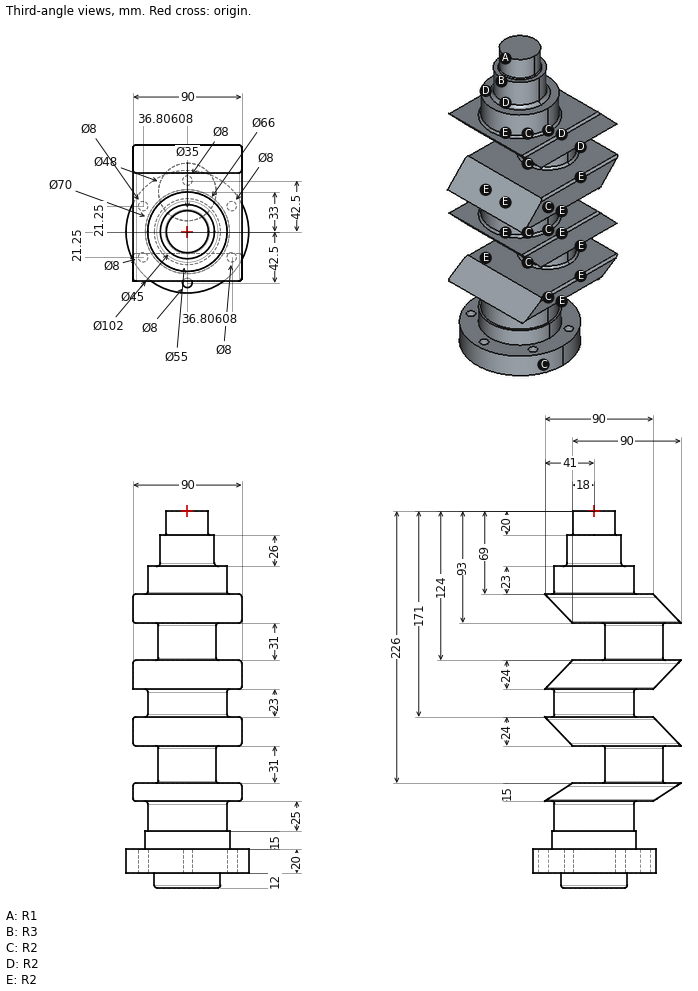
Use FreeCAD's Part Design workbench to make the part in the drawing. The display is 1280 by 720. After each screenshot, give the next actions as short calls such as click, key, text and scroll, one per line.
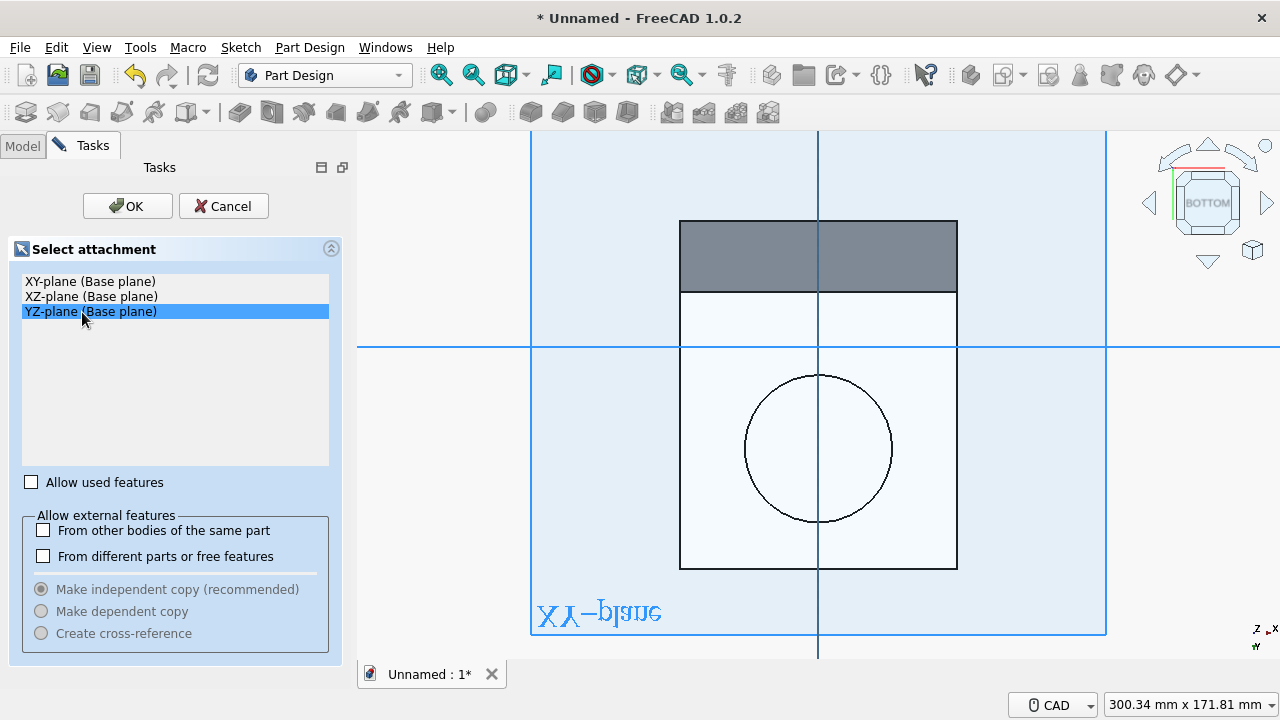
click(128, 206)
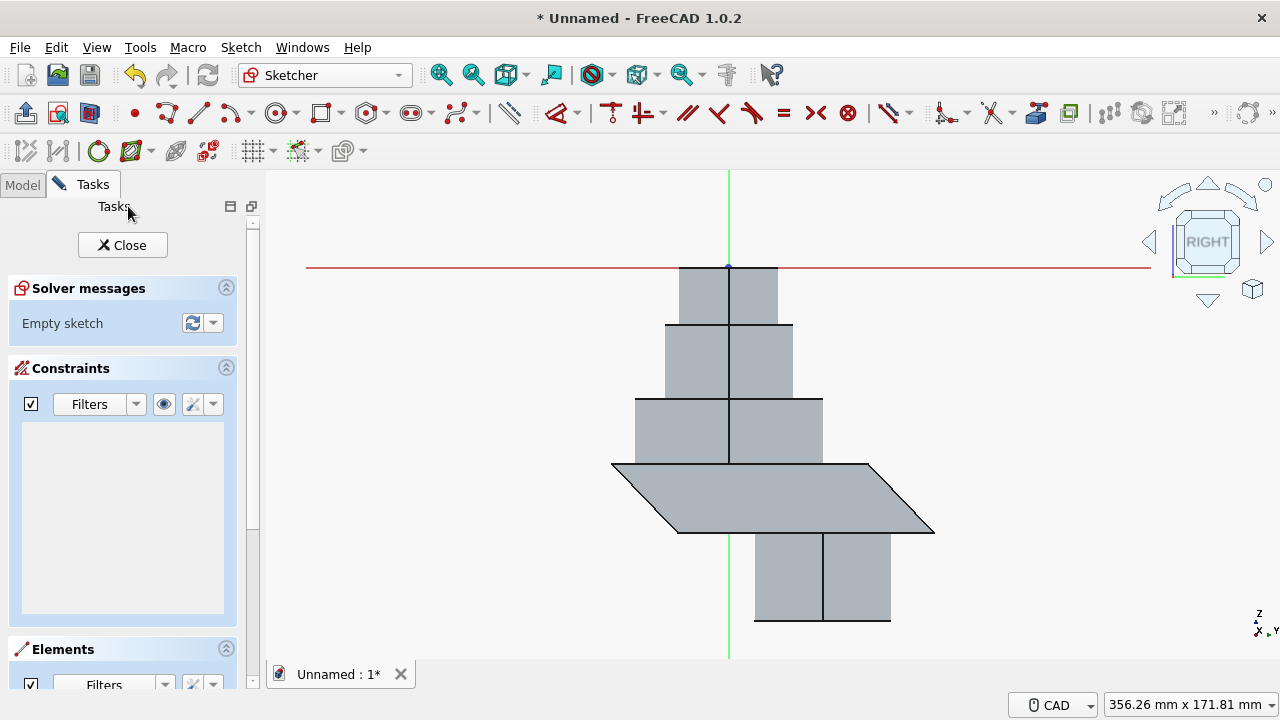
click(90, 114)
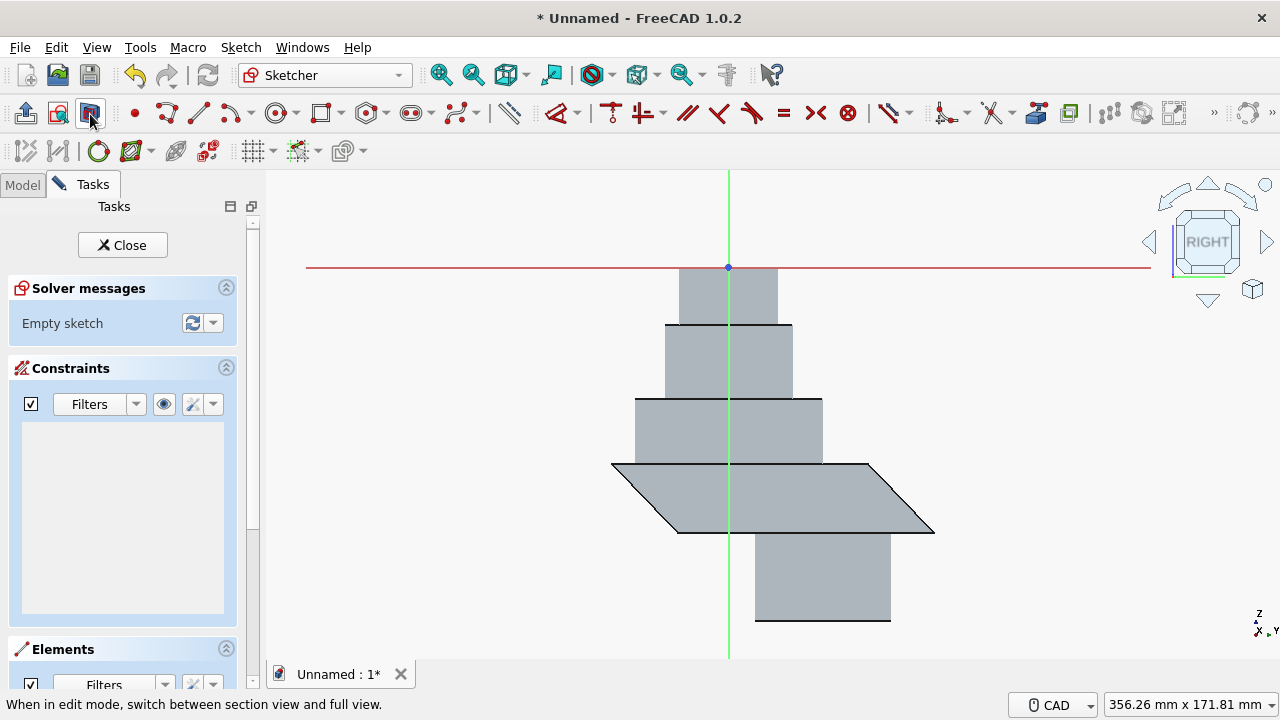
scroll(565, 284, down, 2)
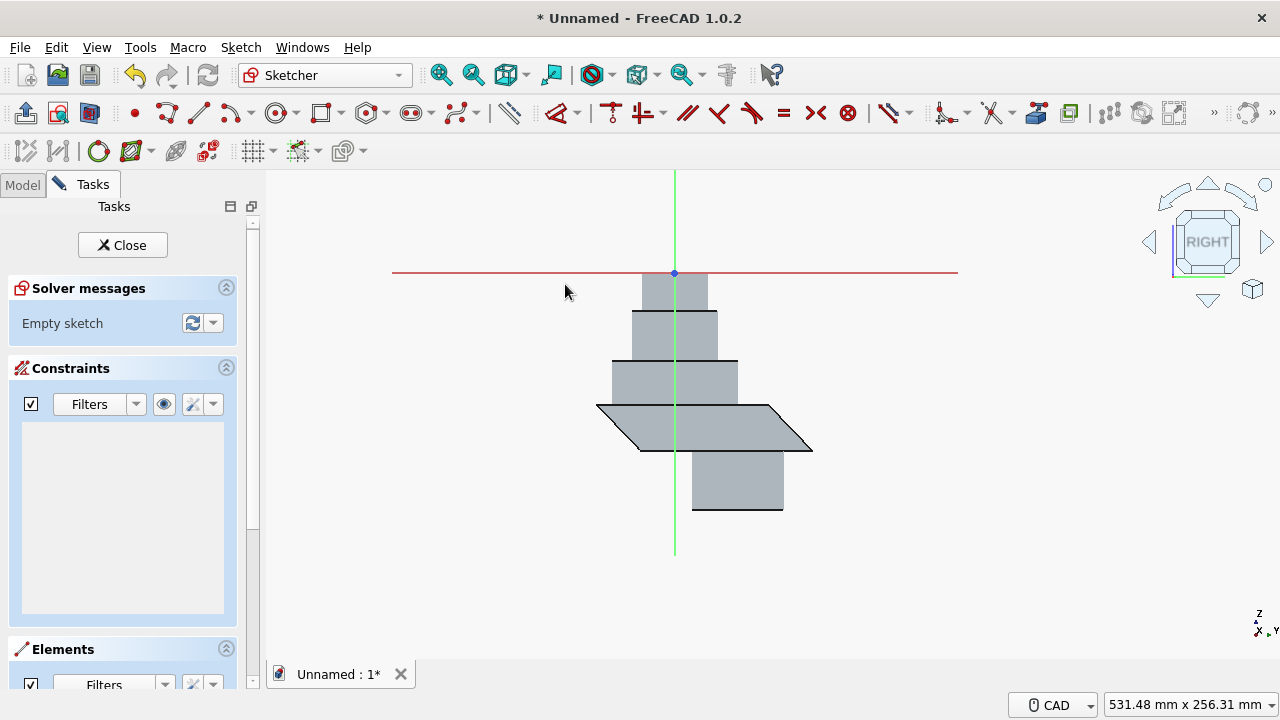
click(168, 114)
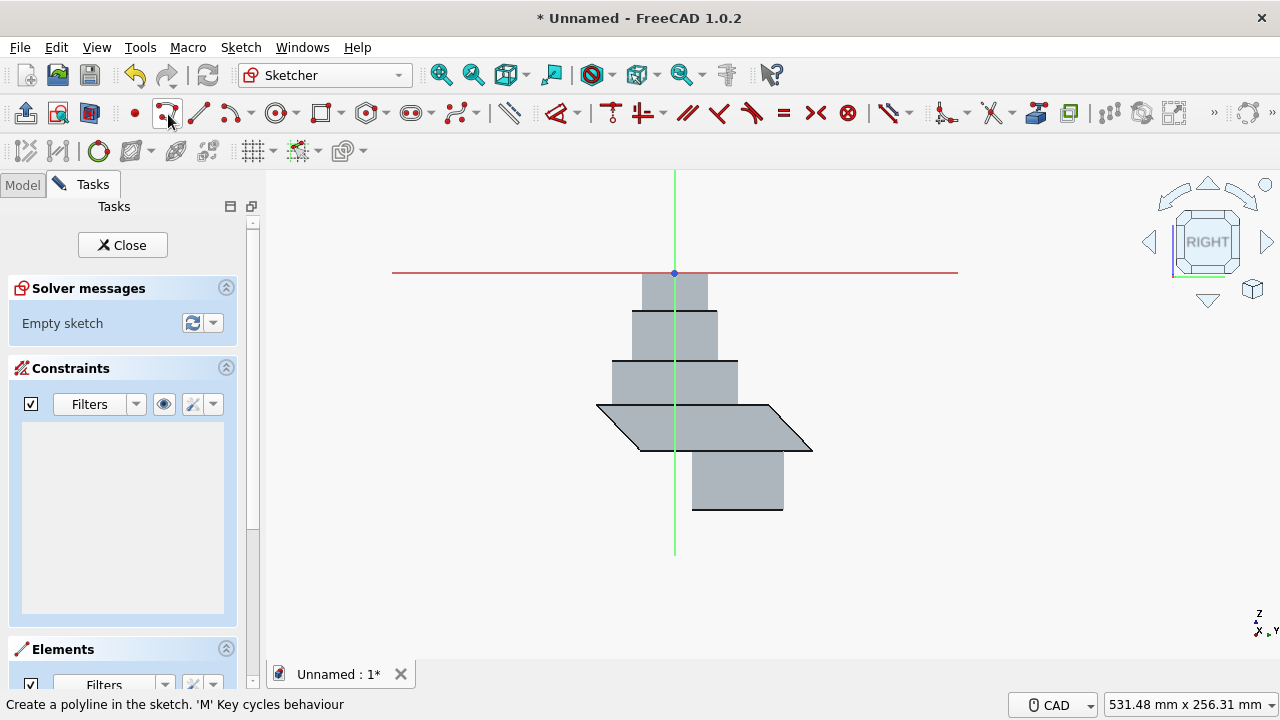
click(641, 510)
click(597, 556)
click(768, 556)
click(812, 510)
click(641, 511)
key(Escape)
key(Escape)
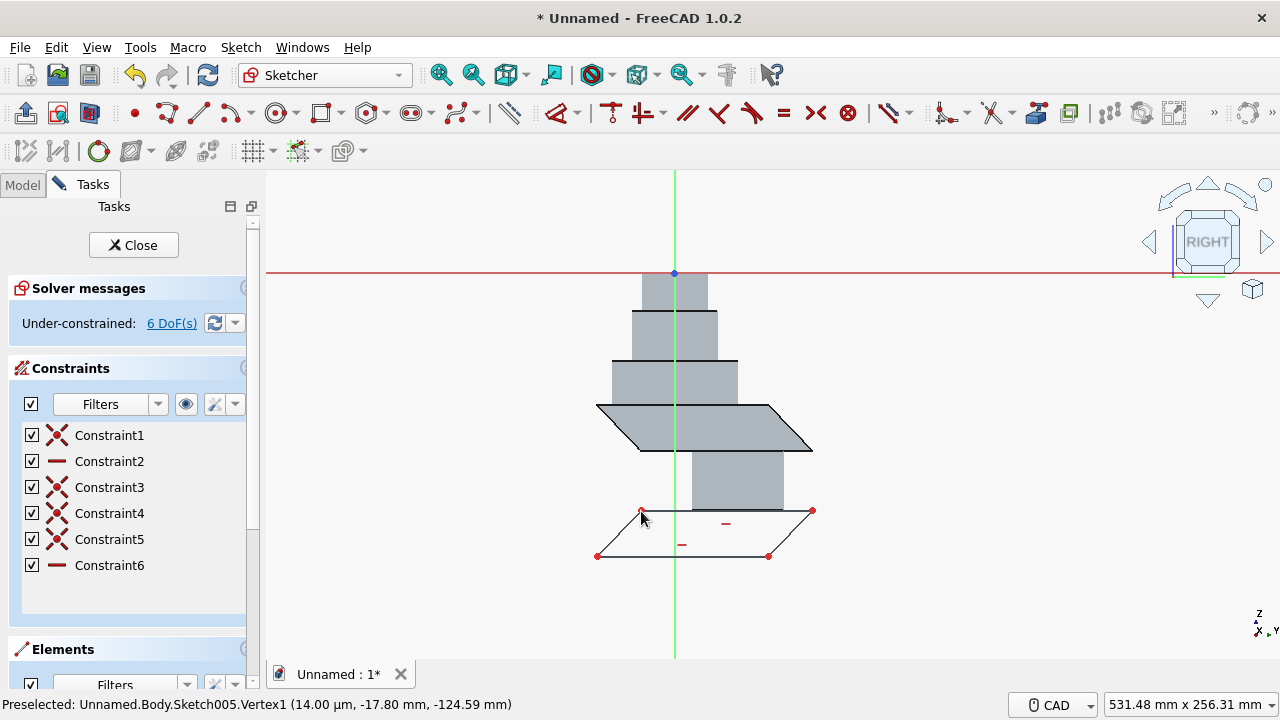
click(556, 114)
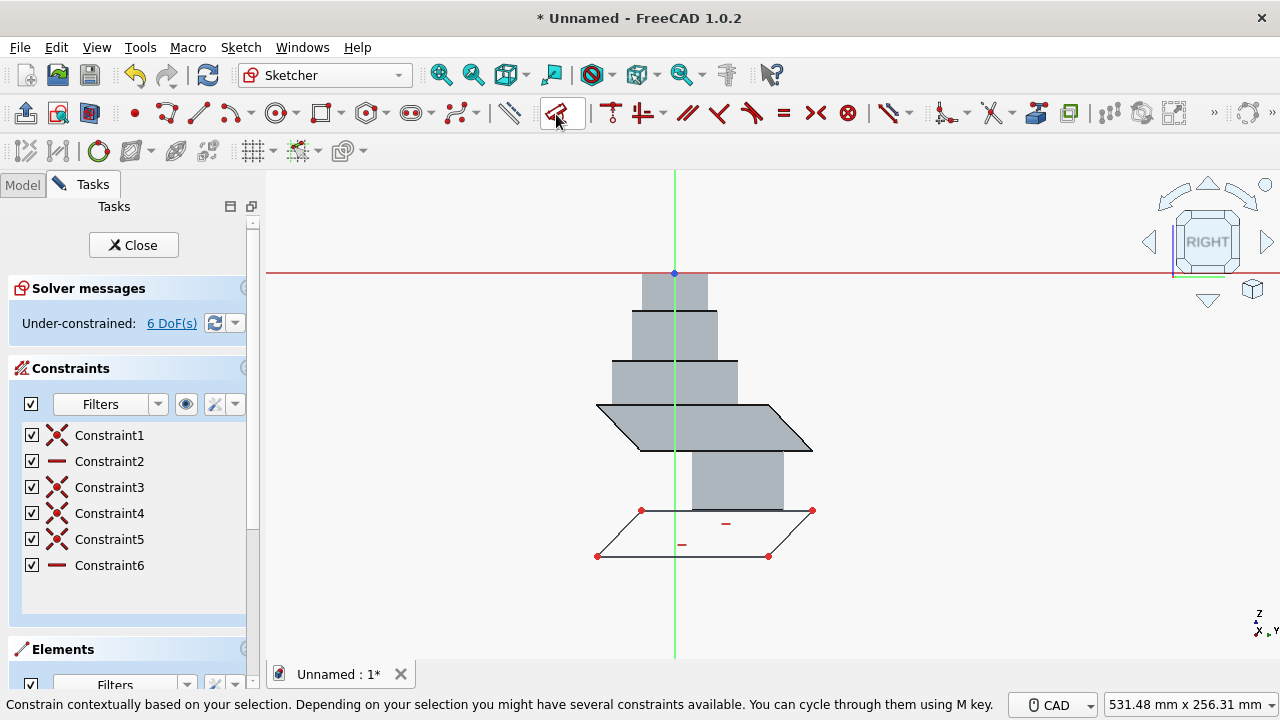
click(648, 557)
click(643, 591)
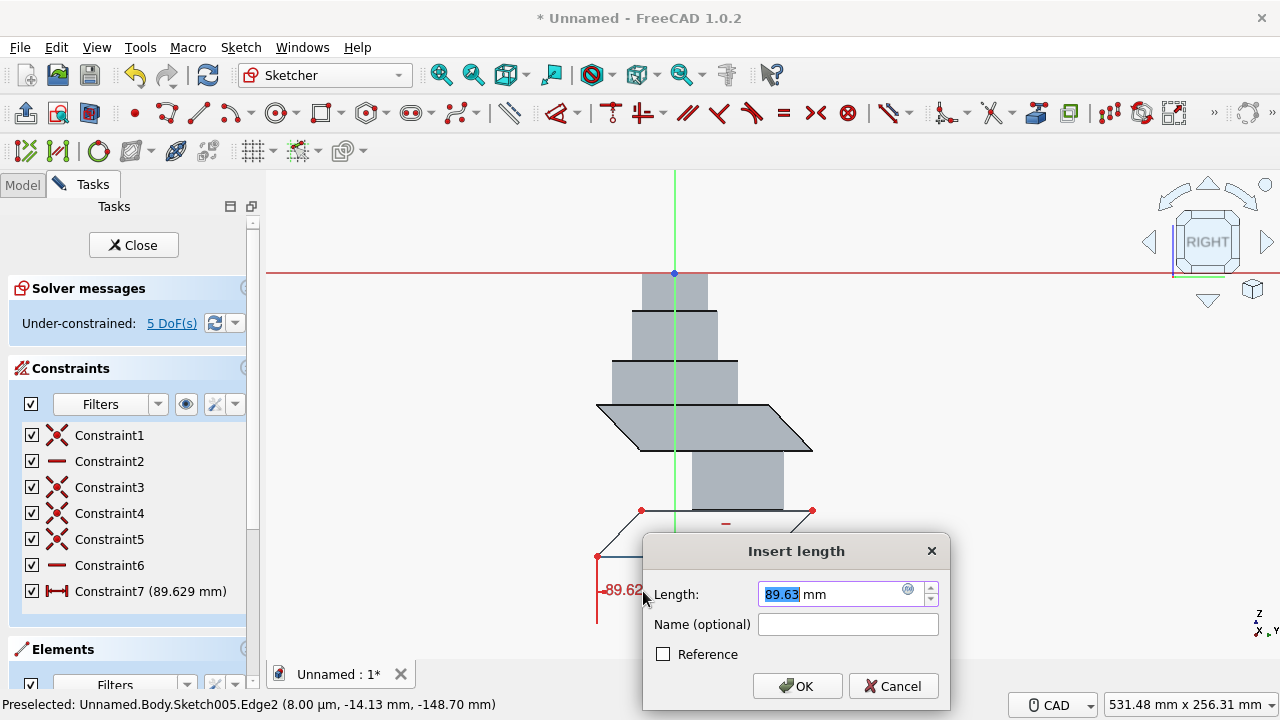
text(90)
key(Return)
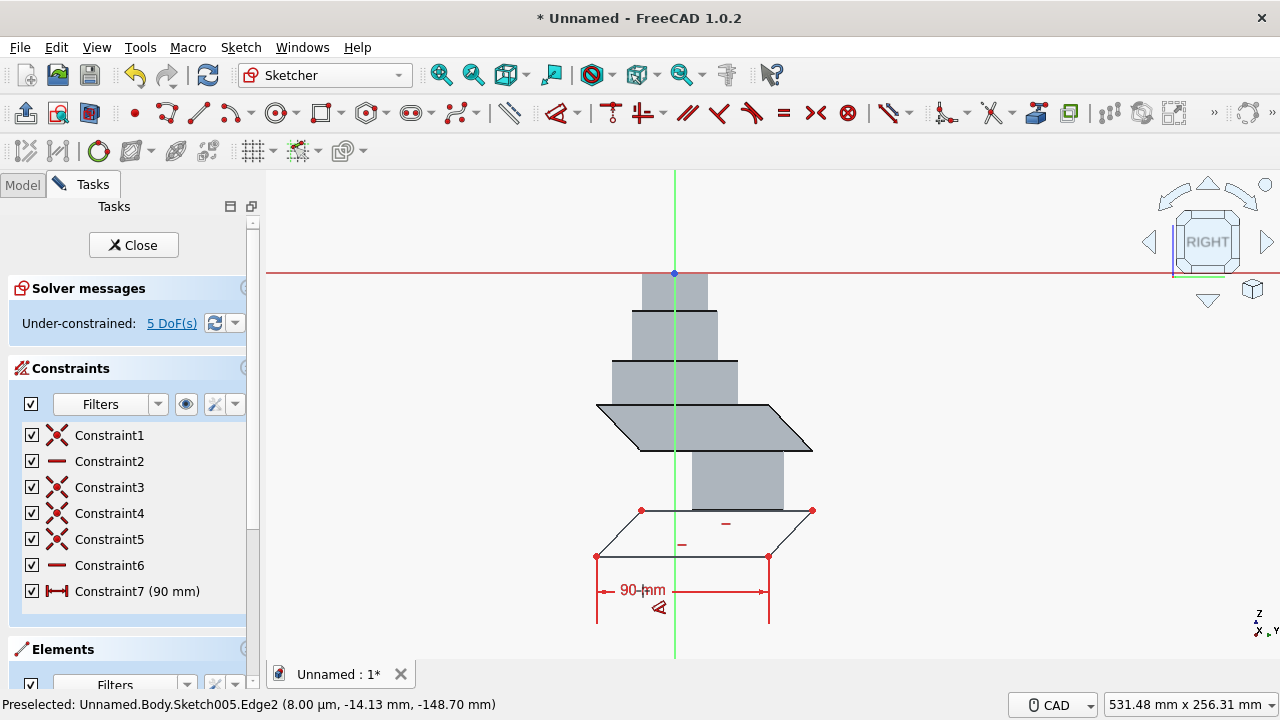
click(761, 511)
click(727, 477)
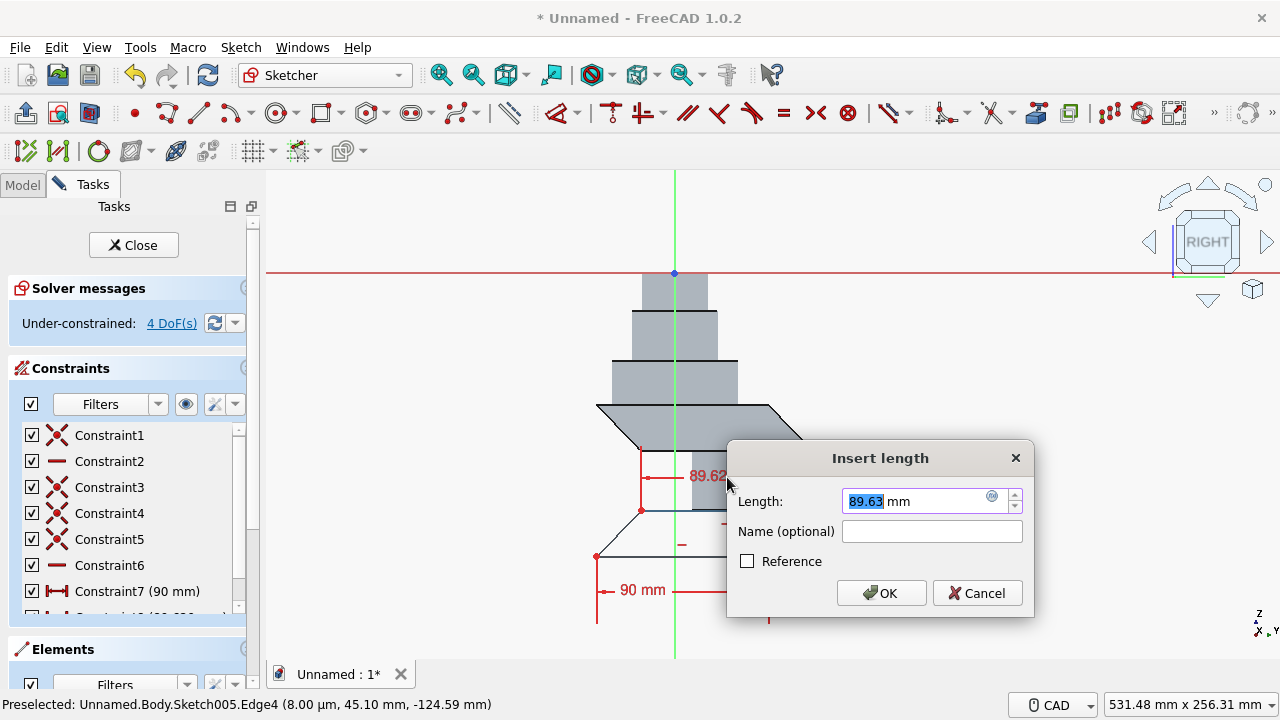
text(90)
key(Return)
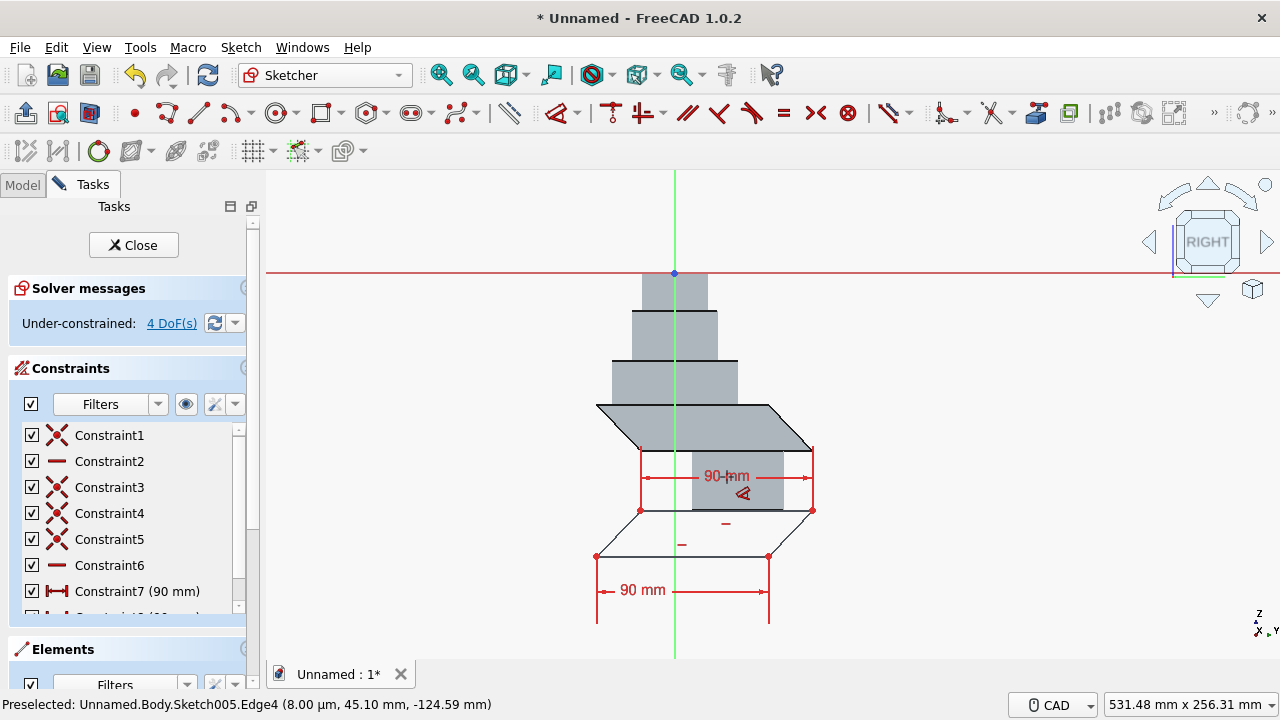
click(641, 511)
click(658, 239)